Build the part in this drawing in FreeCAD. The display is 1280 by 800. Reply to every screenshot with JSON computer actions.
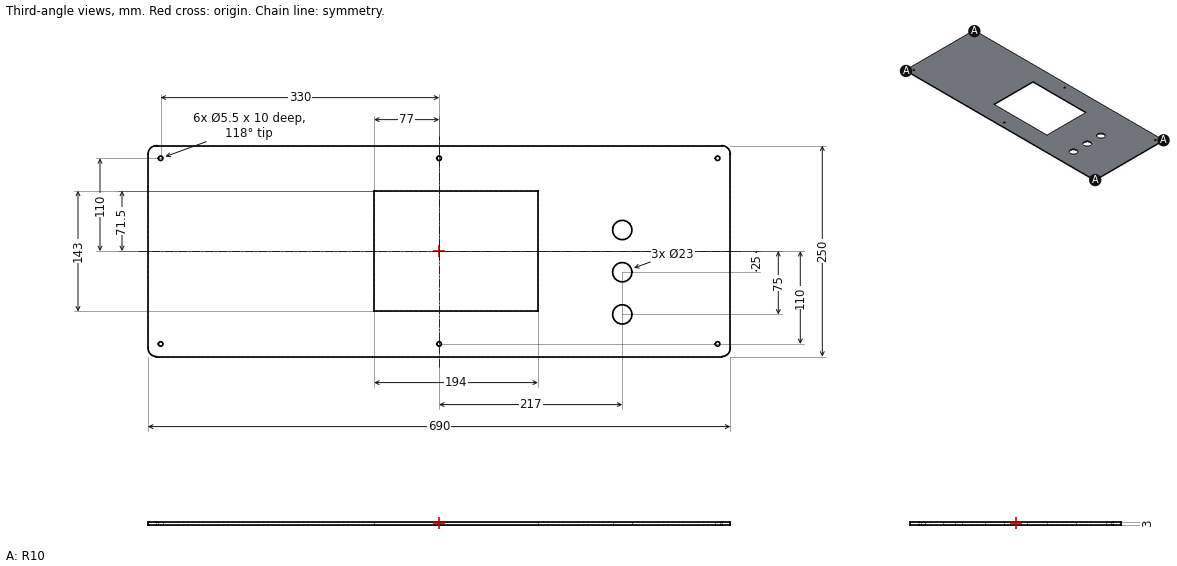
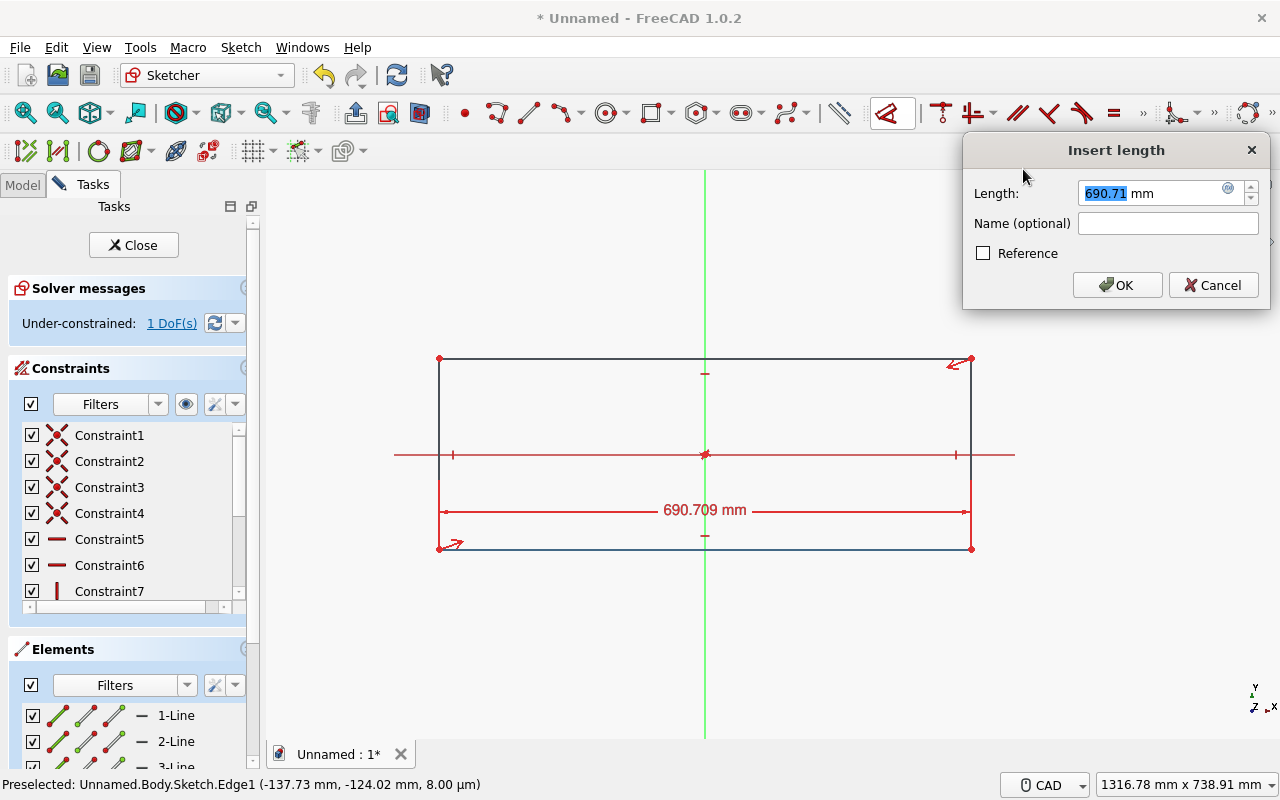
{"action": "type", "text": "690"}
{"action": "key", "text": "Return"}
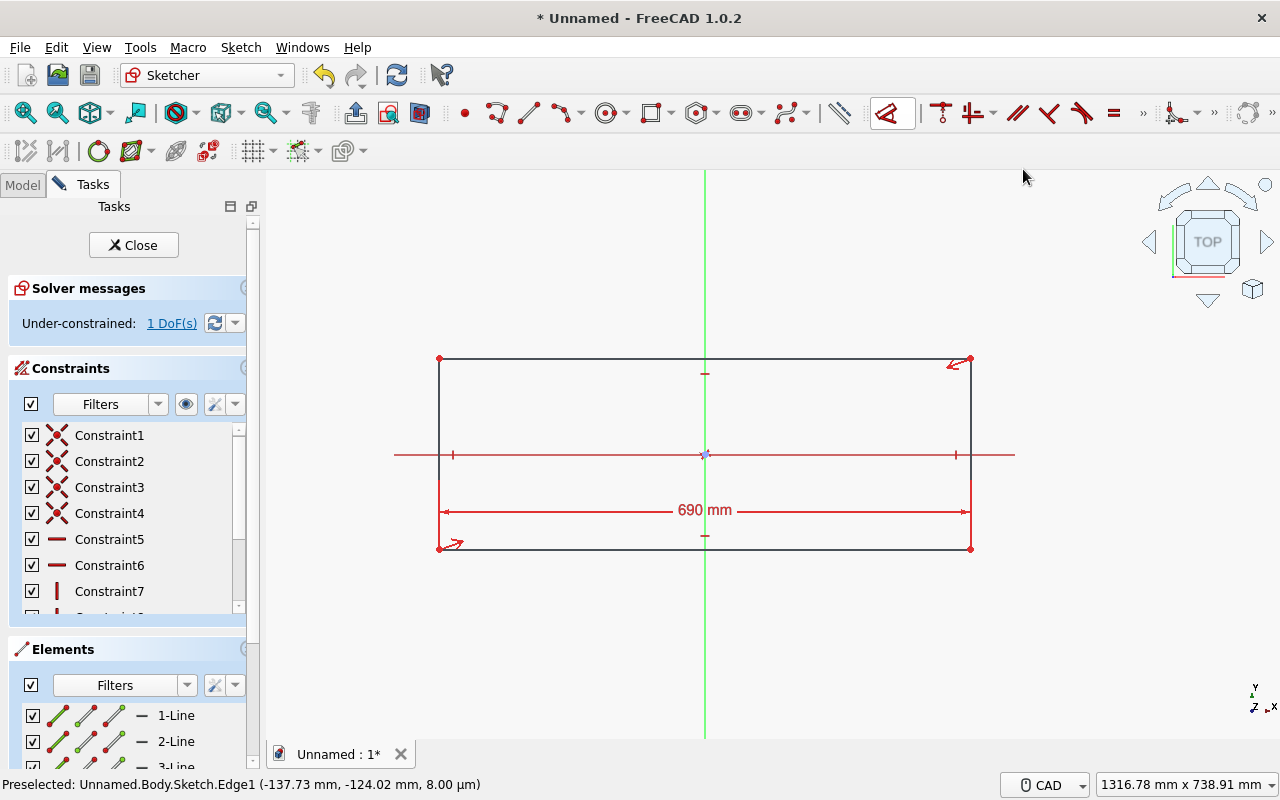
{"action": "left_click", "coordinate": [971, 493]}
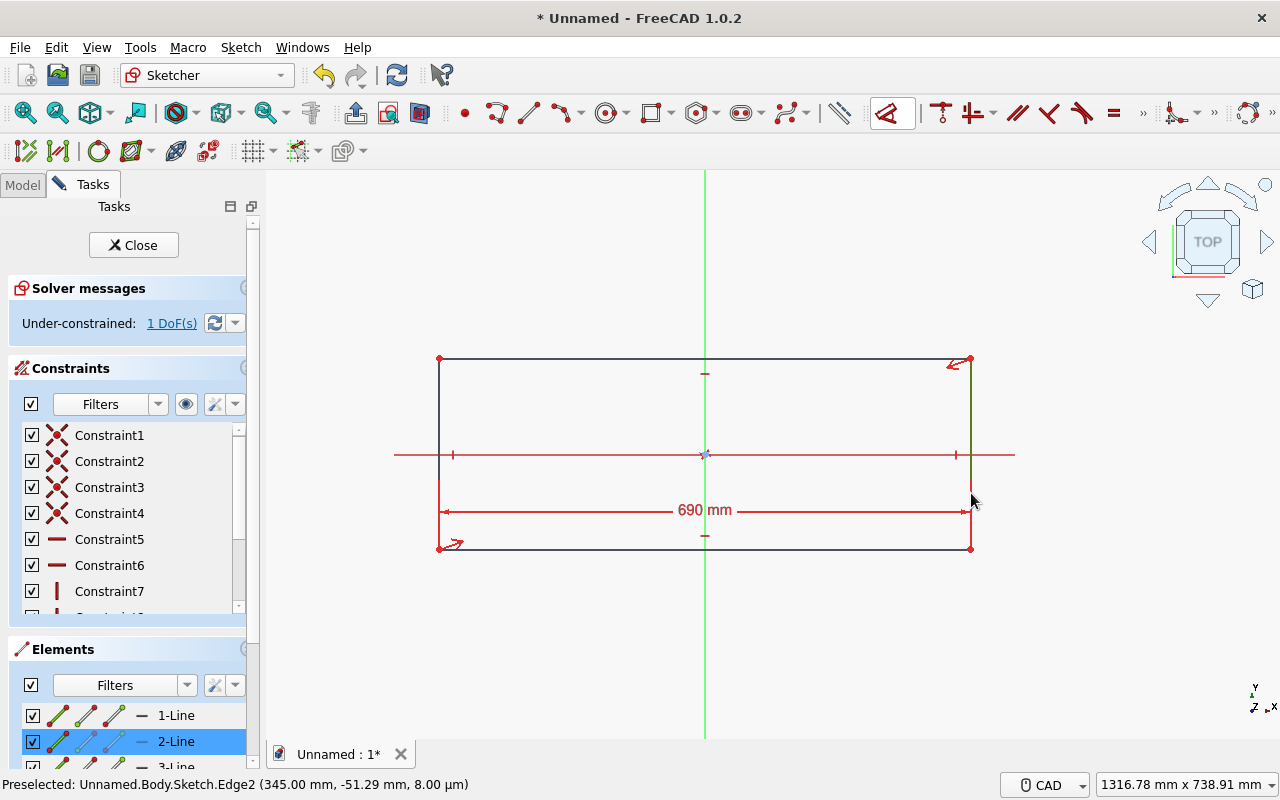
{"action": "key", "text": "i"}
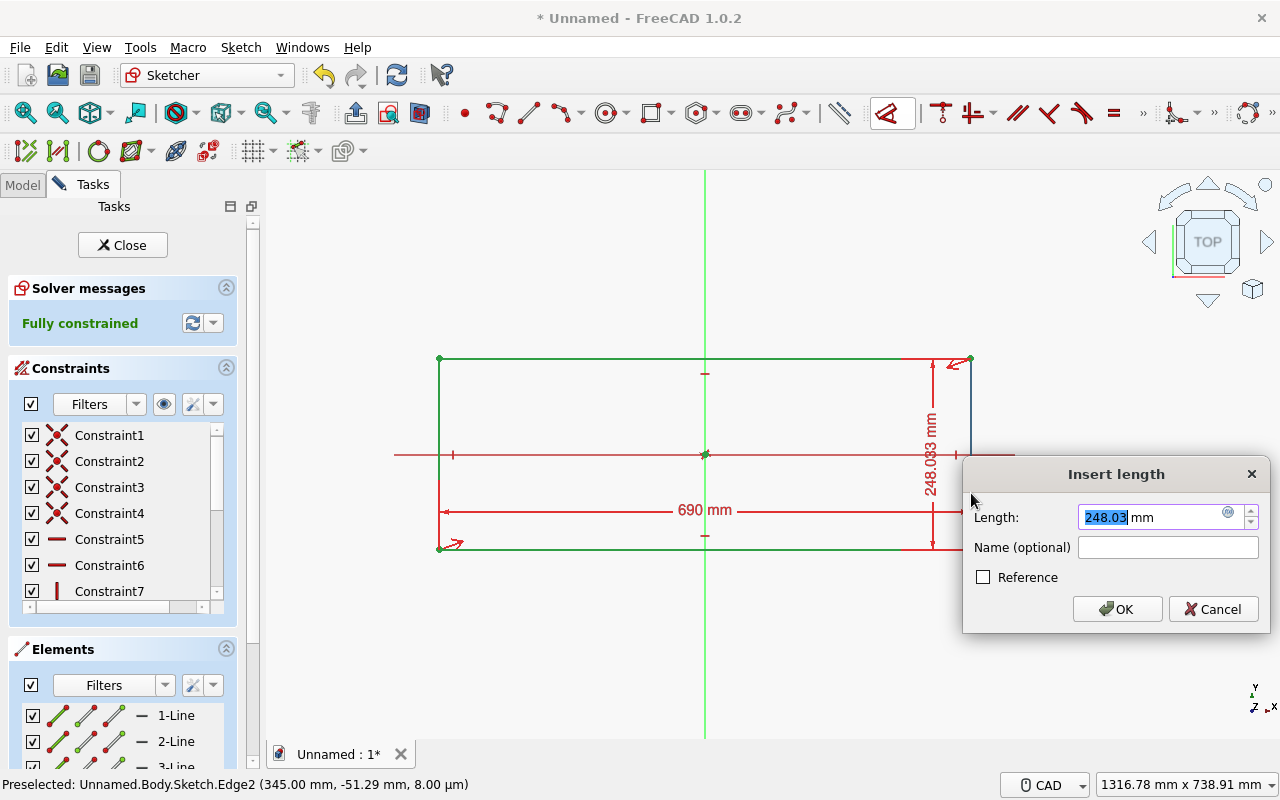
{"action": "type", "text": "250"}
{"action": "key", "text": "Return"}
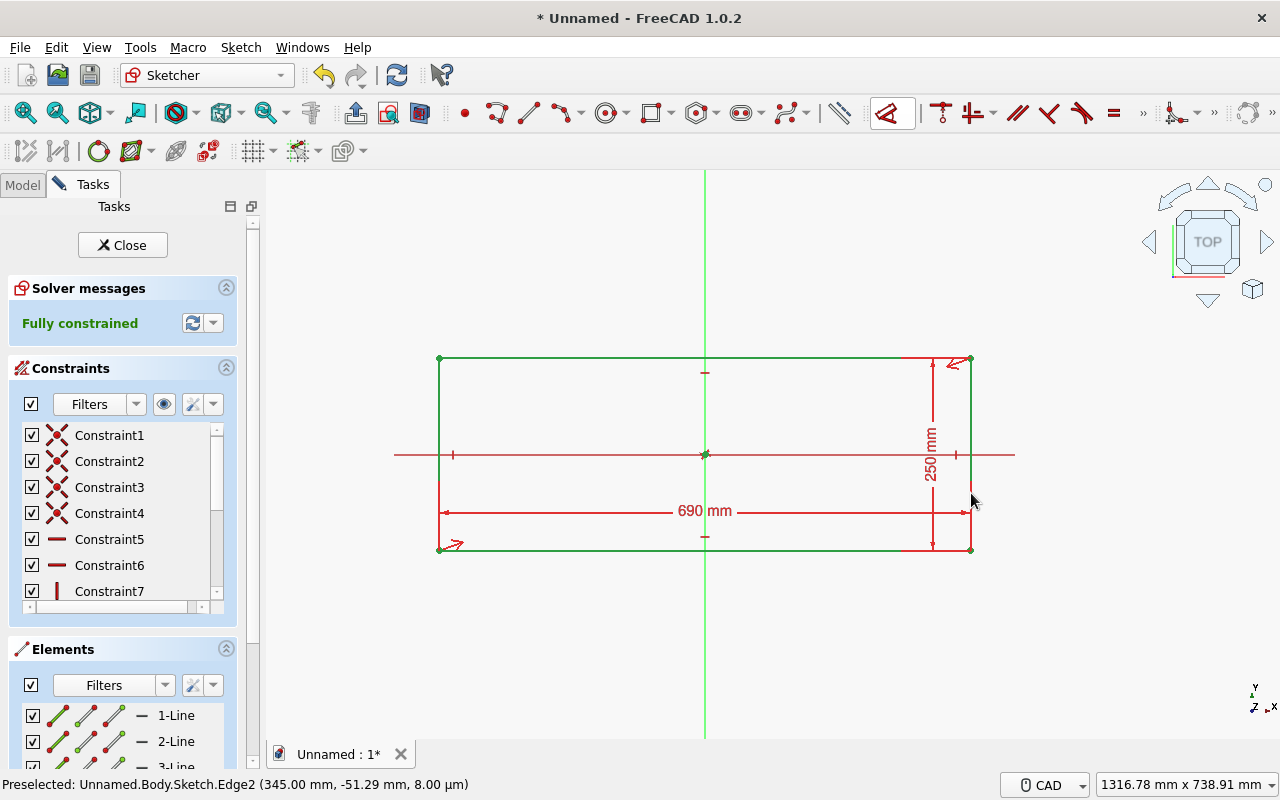
{"action": "left_click", "coordinate": [123, 245]}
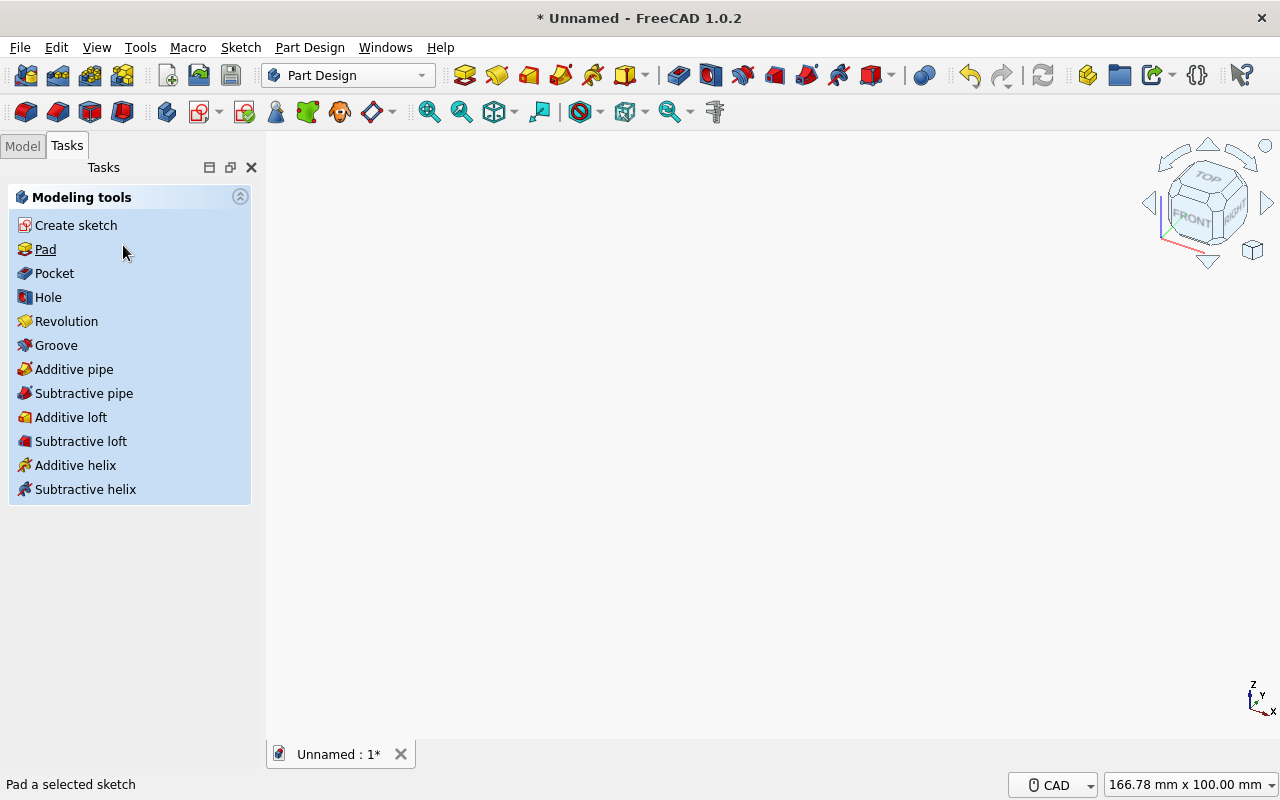
{"action": "left_click", "coordinate": [466, 76]}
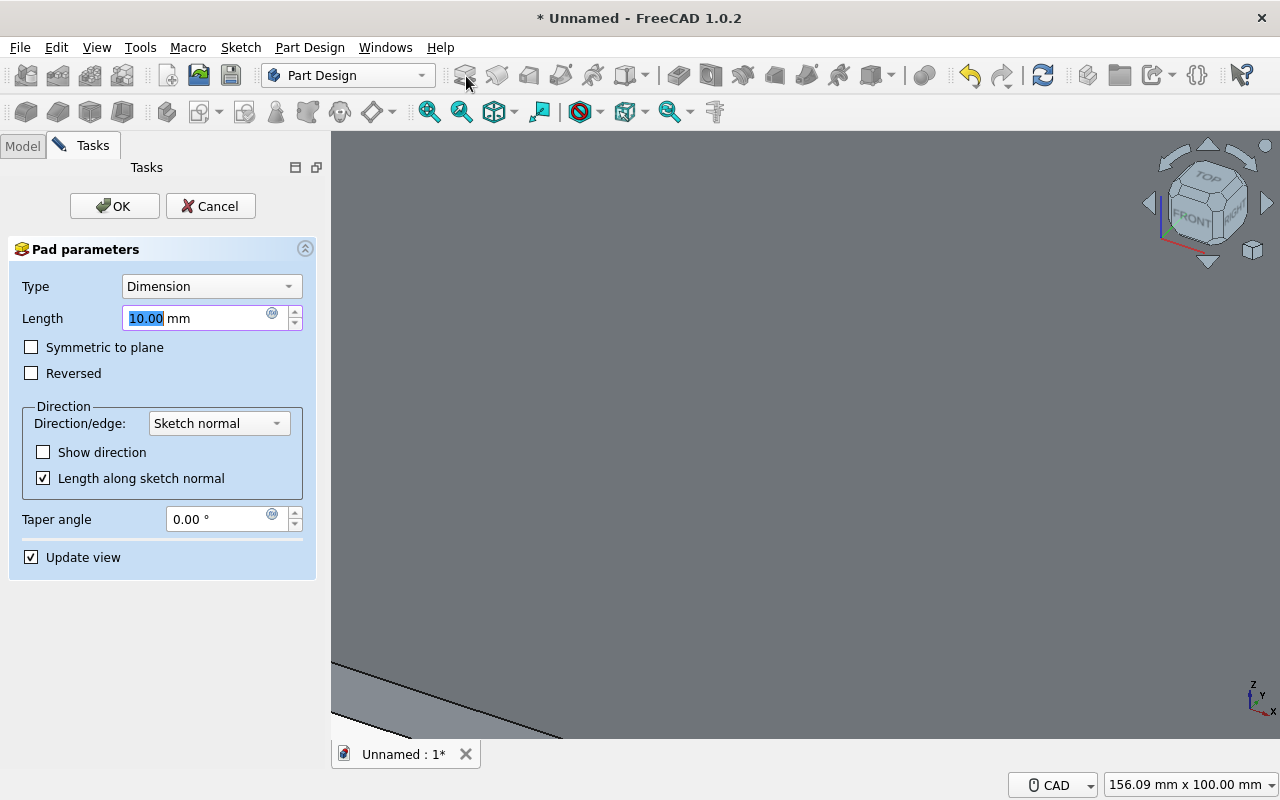
{"action": "type", "text": "3"}
{"action": "key", "text": "Tab"}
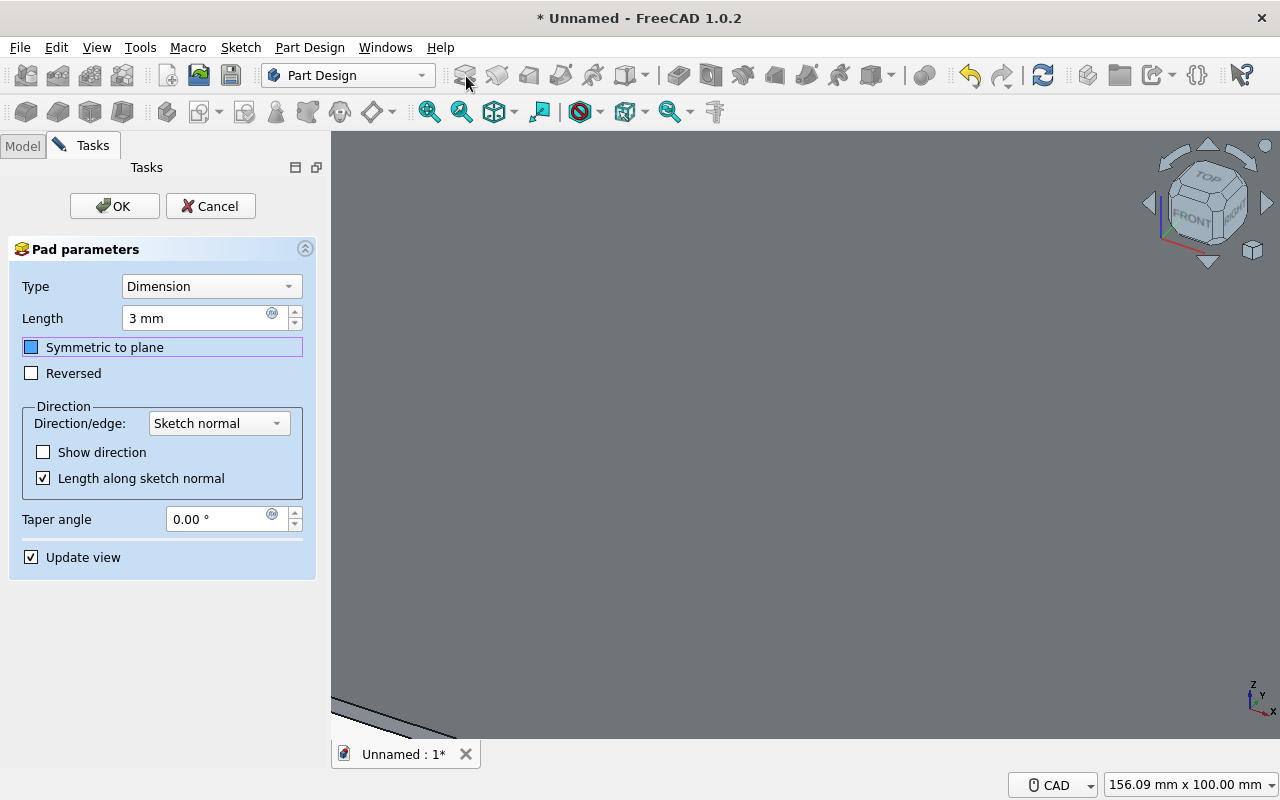
{"action": "left_click", "coordinate": [30, 347]}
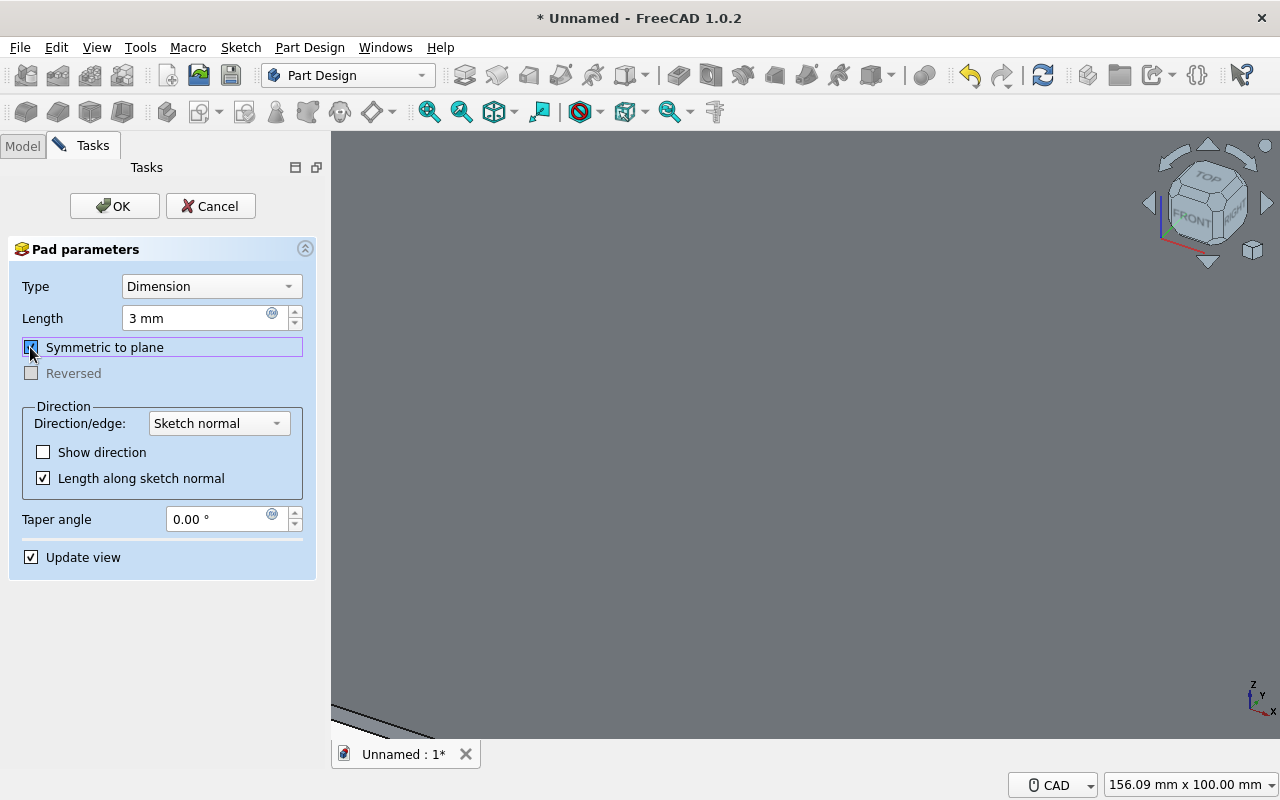
{"action": "left_click", "coordinate": [115, 206]}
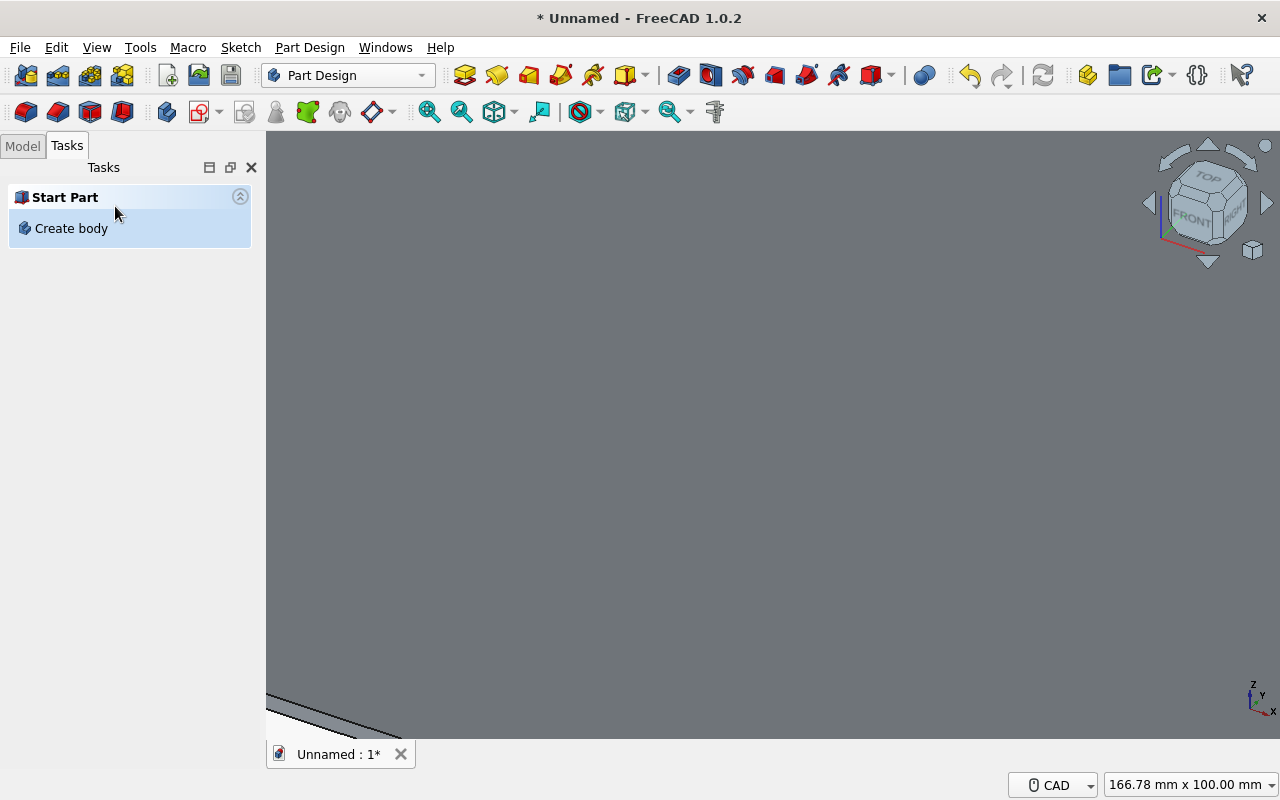
{"action": "left_click", "coordinate": [430, 112]}